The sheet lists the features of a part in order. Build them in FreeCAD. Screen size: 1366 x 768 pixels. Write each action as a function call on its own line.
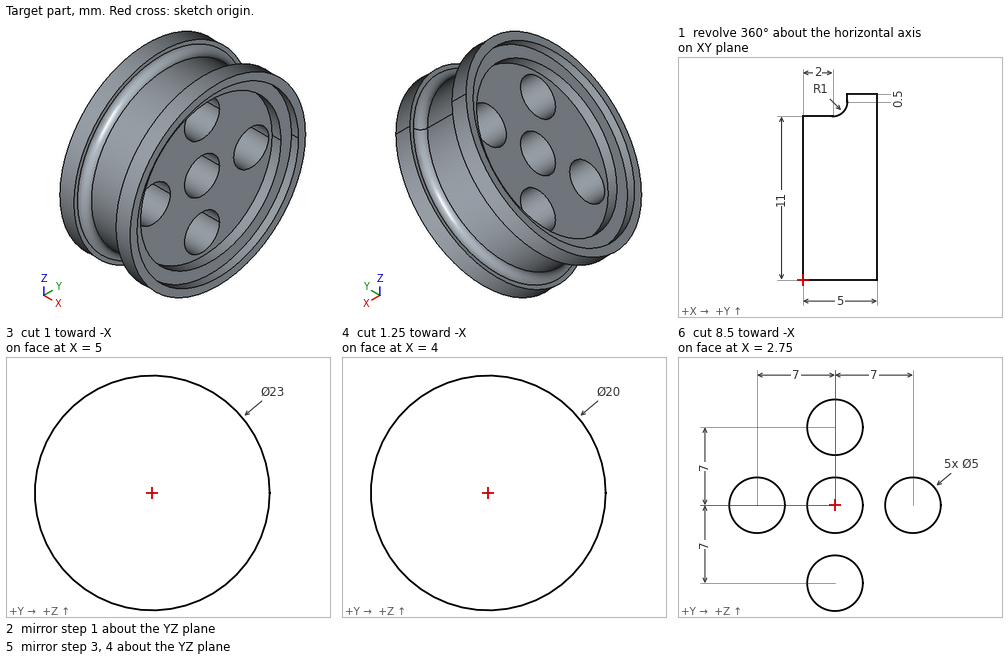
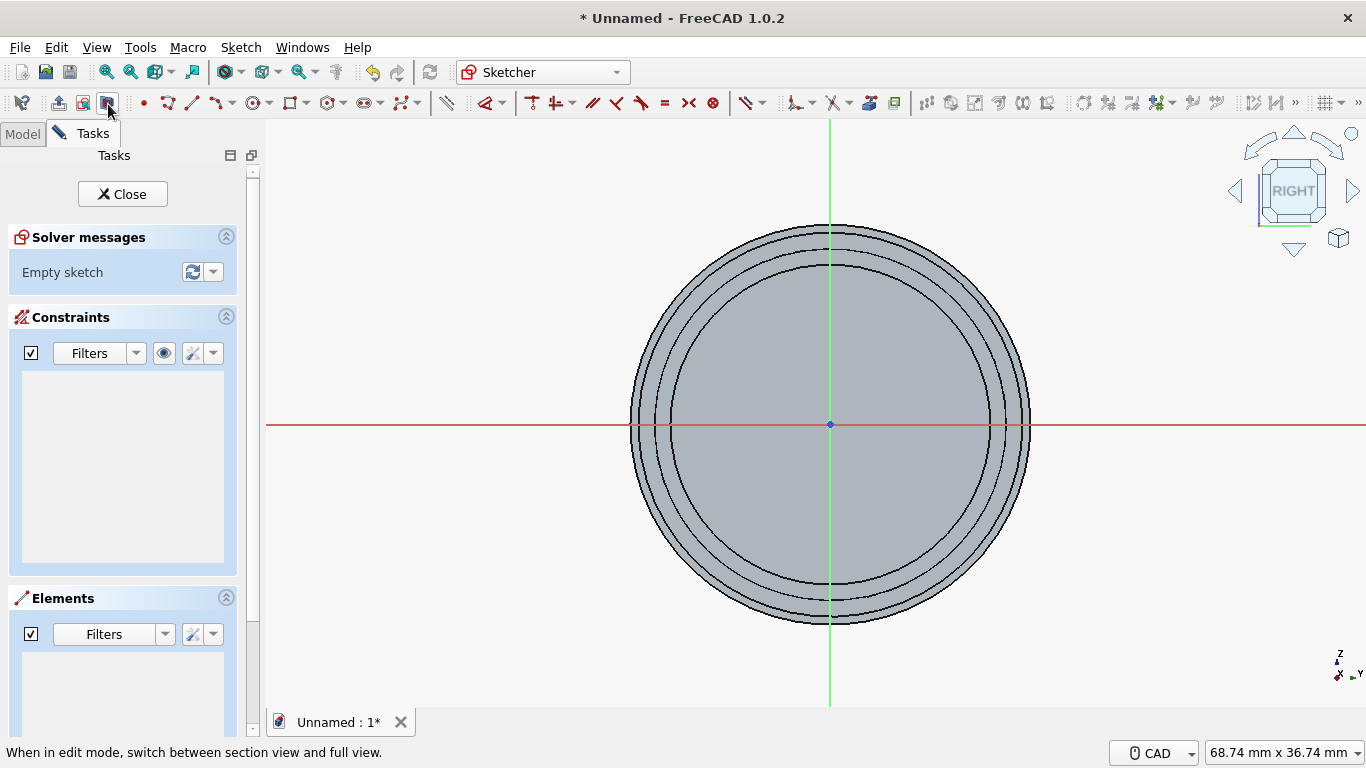
click(254, 104)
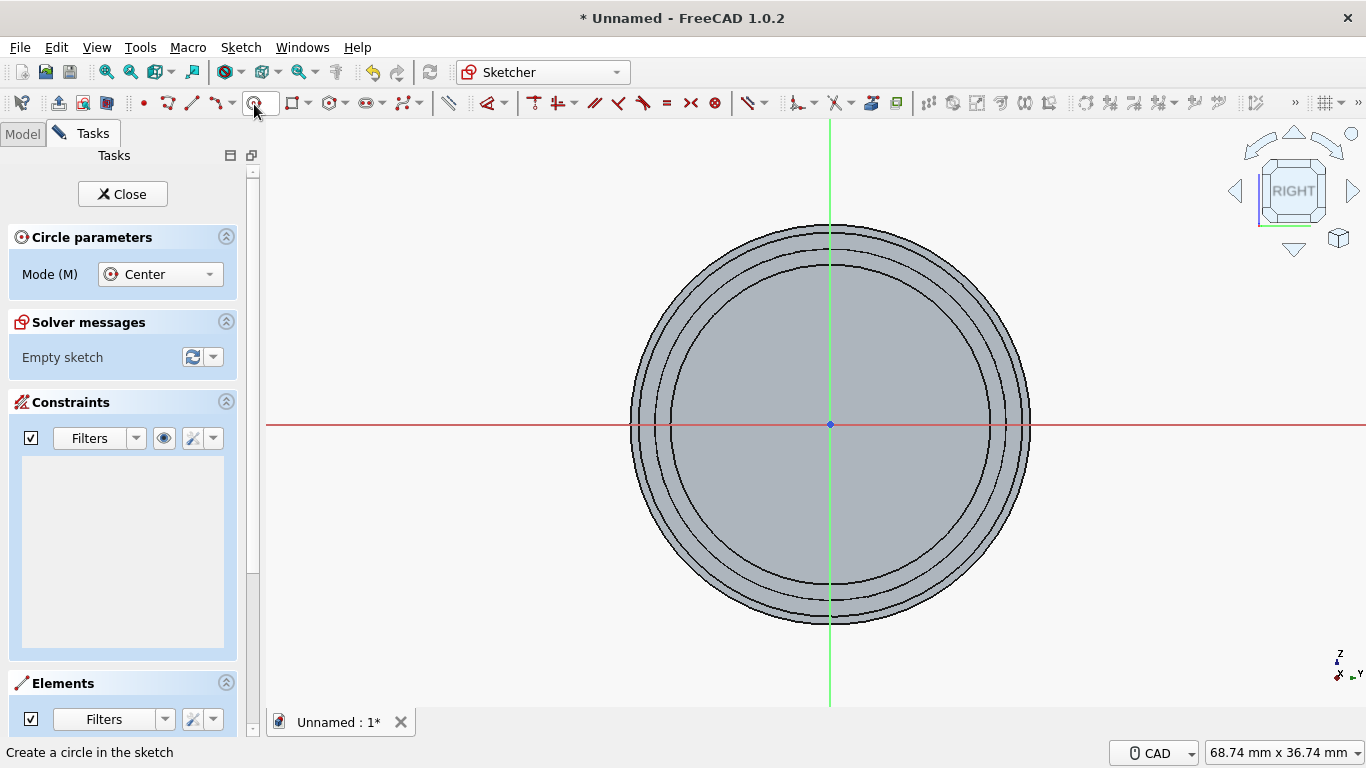
click(942, 425)
click(971, 396)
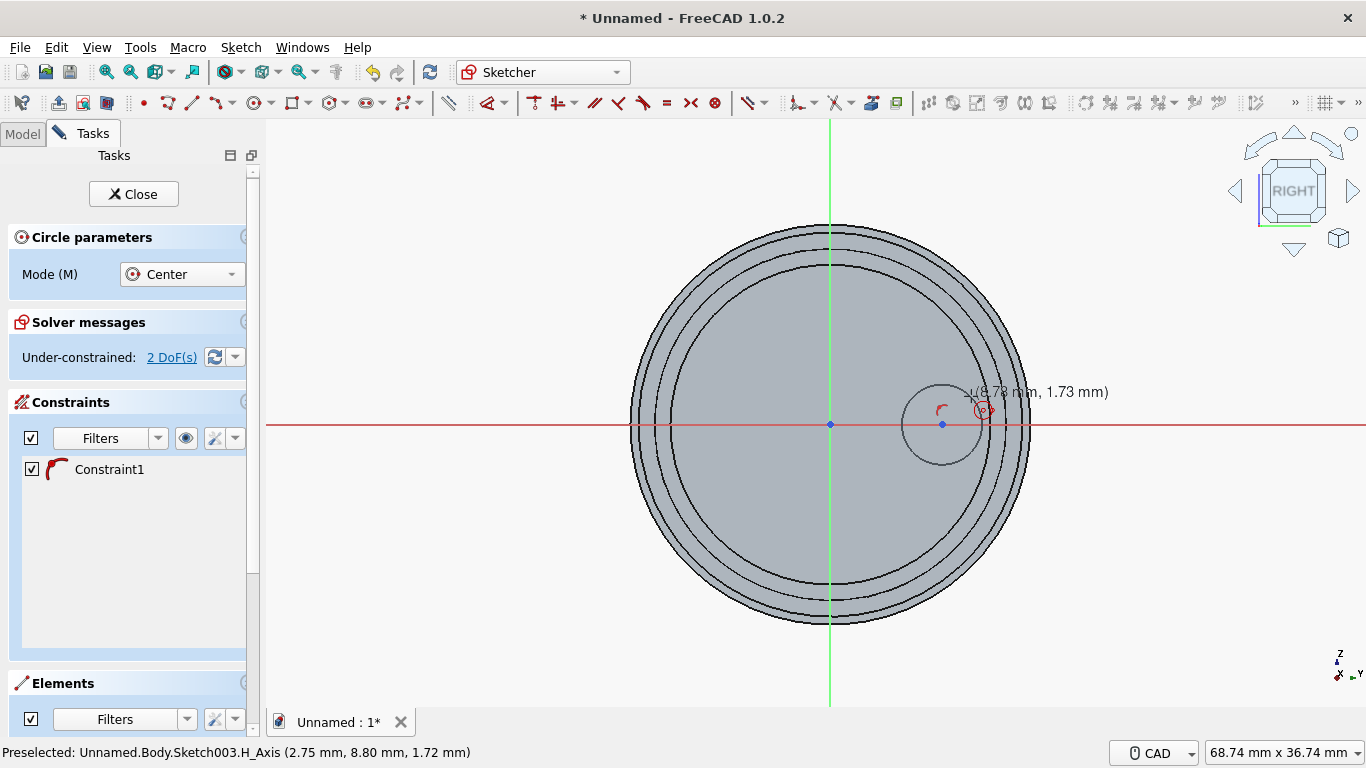
click(830, 537)
click(859, 508)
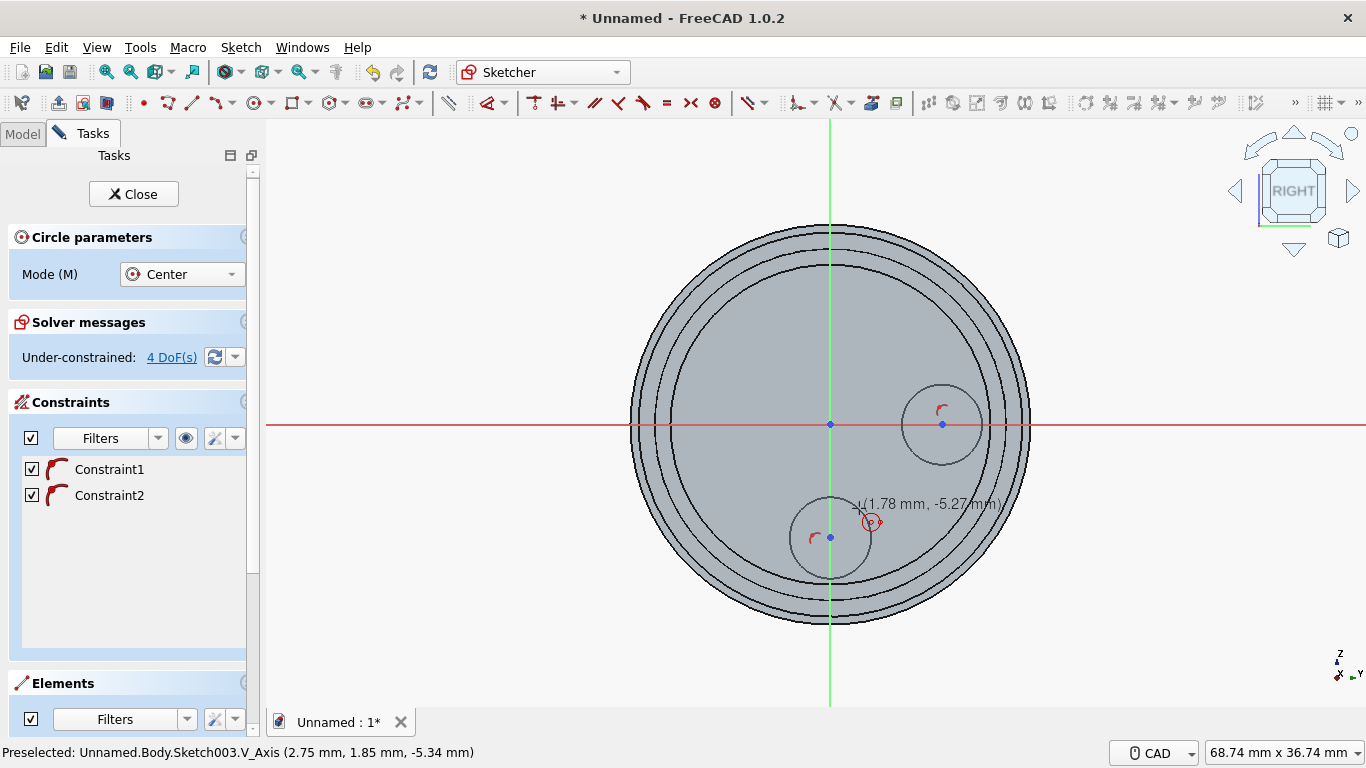
click(718, 425)
click(747, 396)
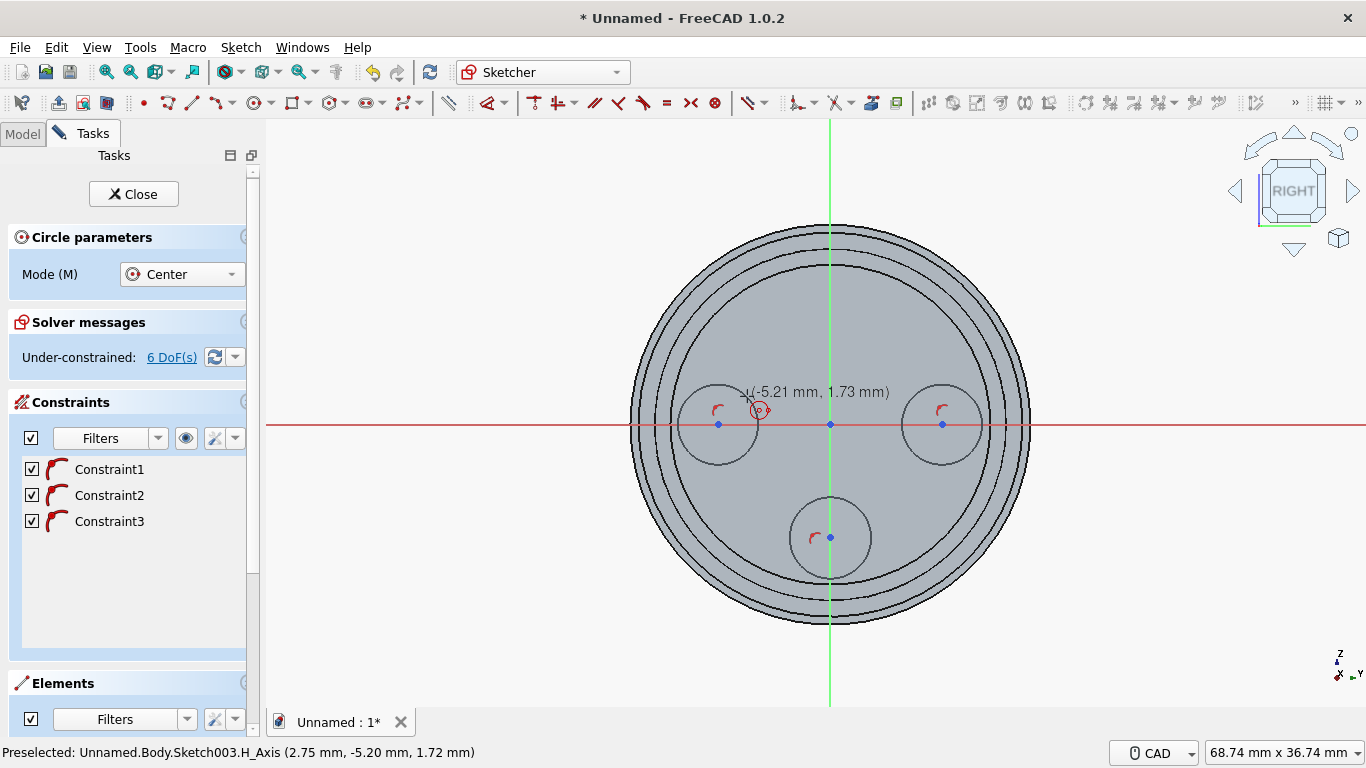
click(830, 313)
click(859, 284)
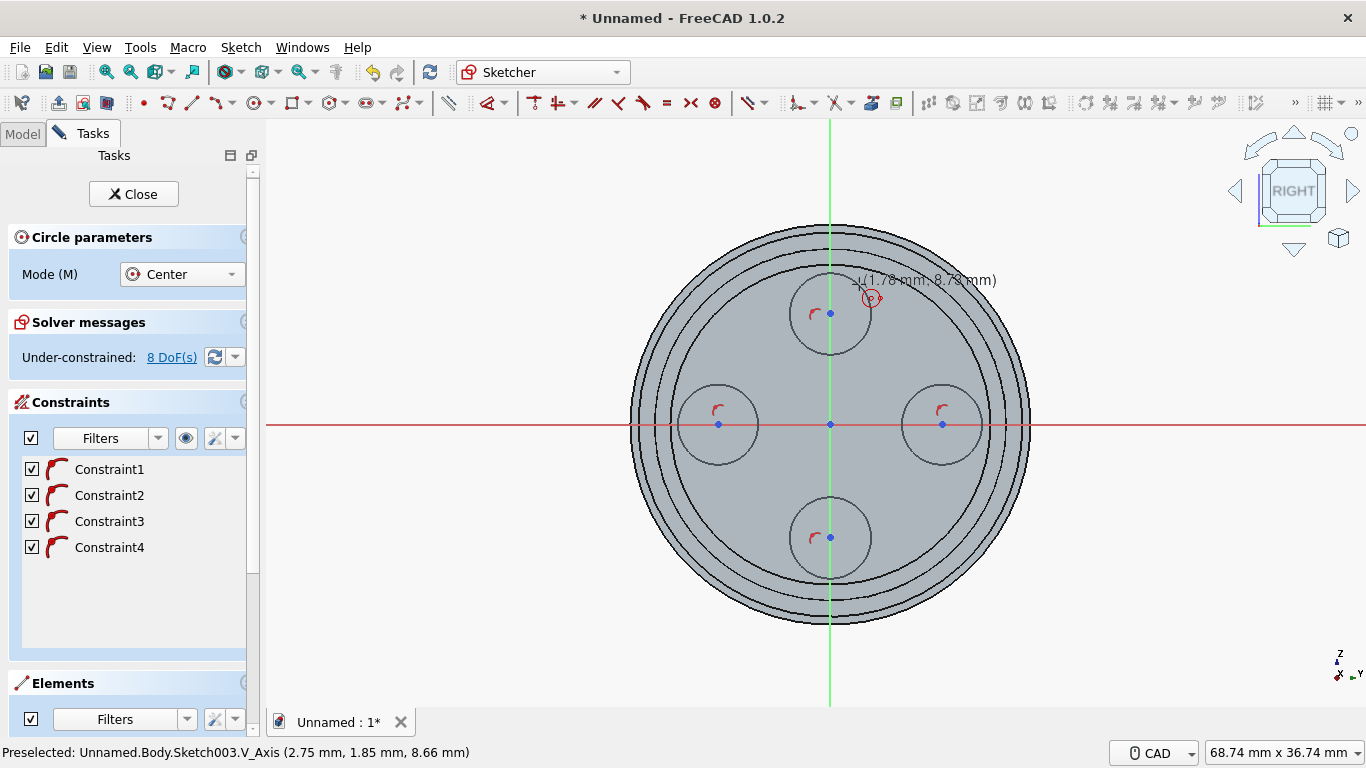
click(830, 425)
click(859, 396)
key(Escape)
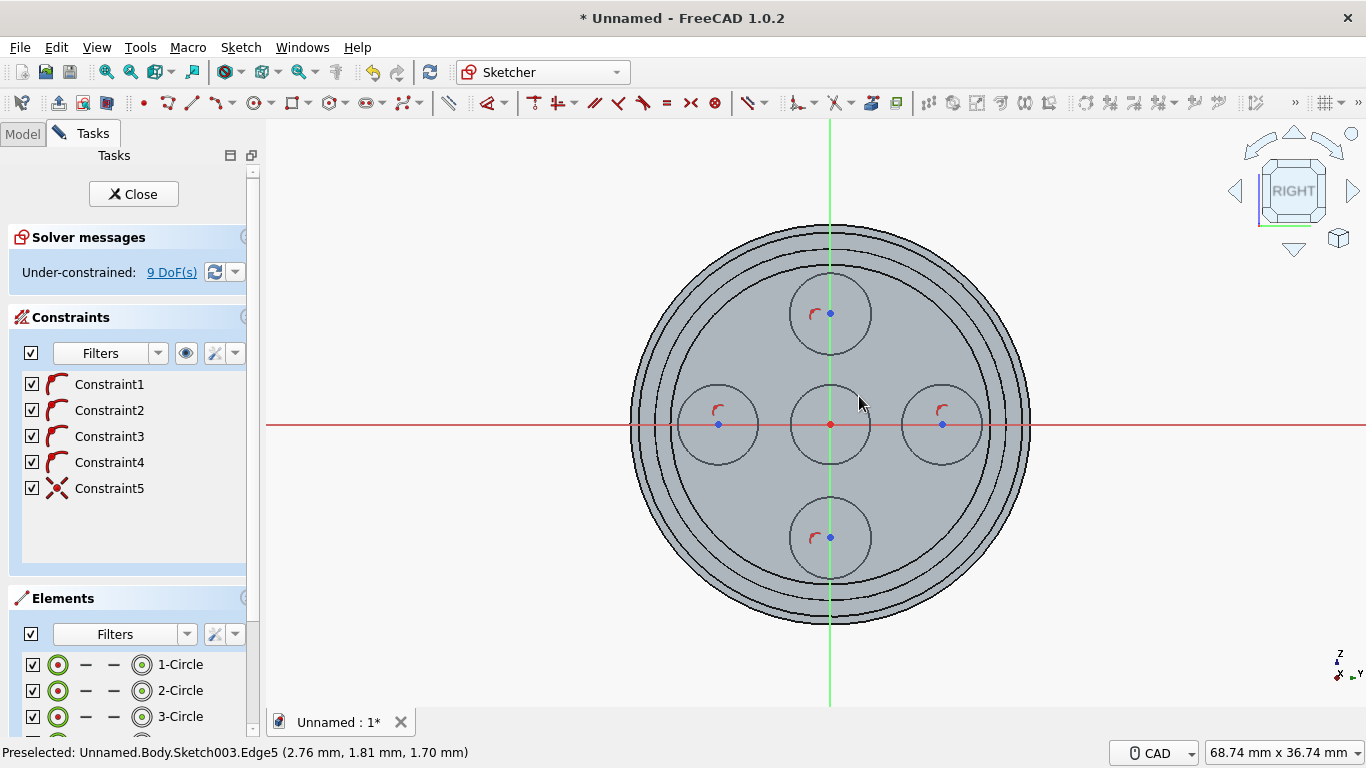
click(970, 396)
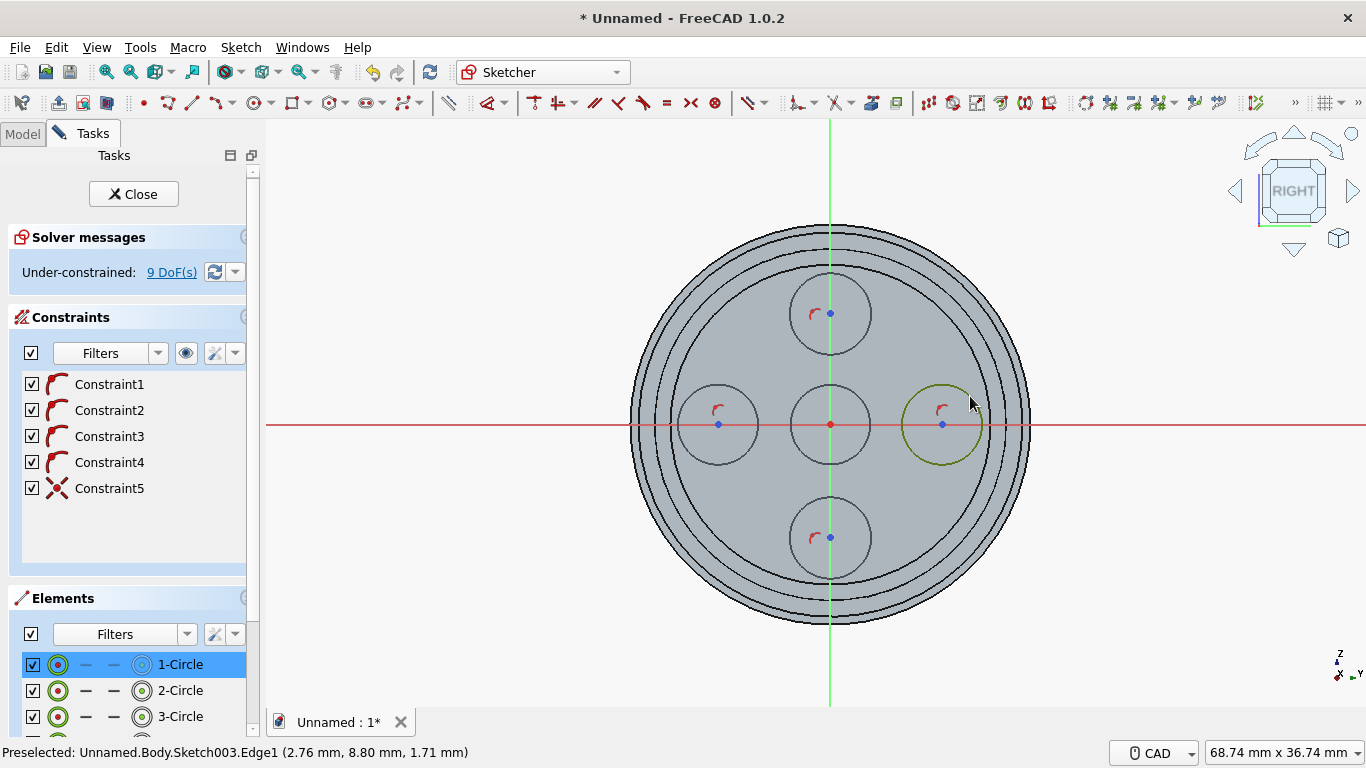
click(859, 509)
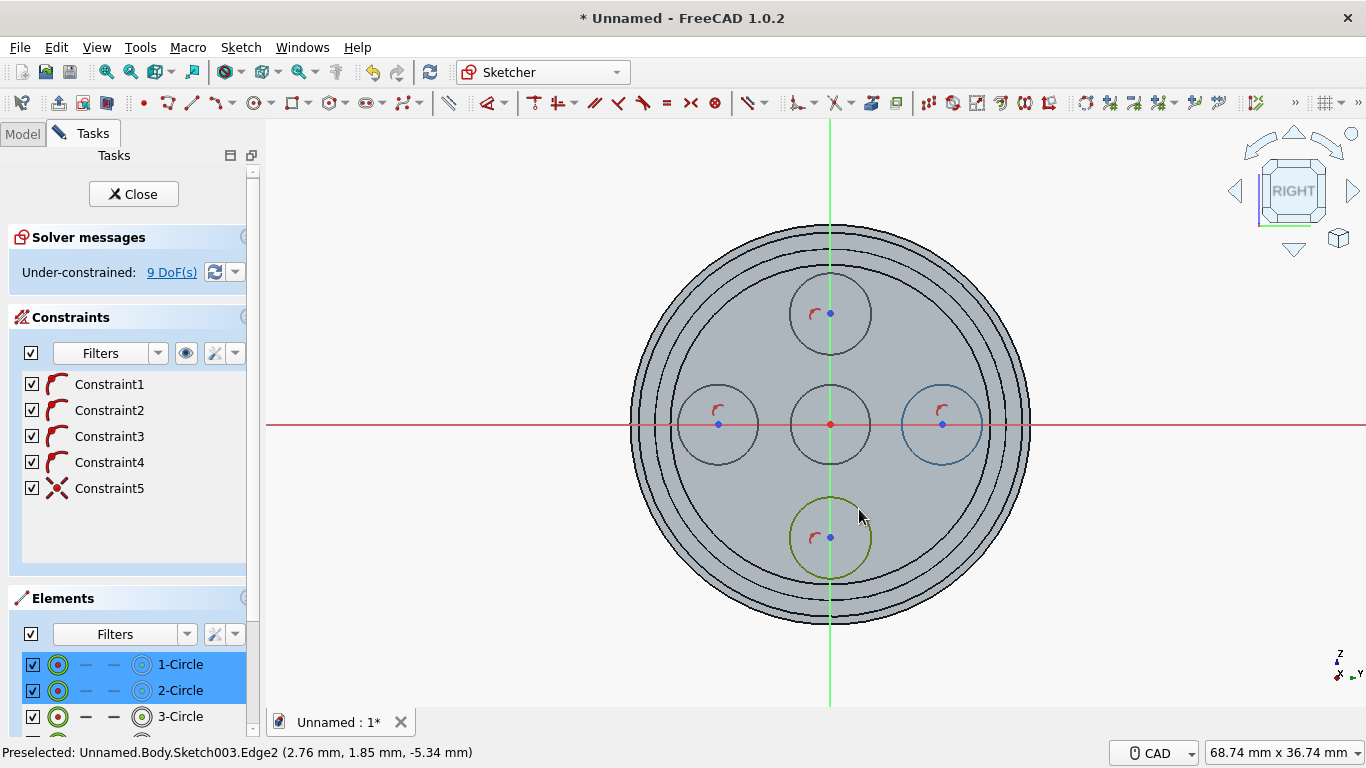
click(746, 396)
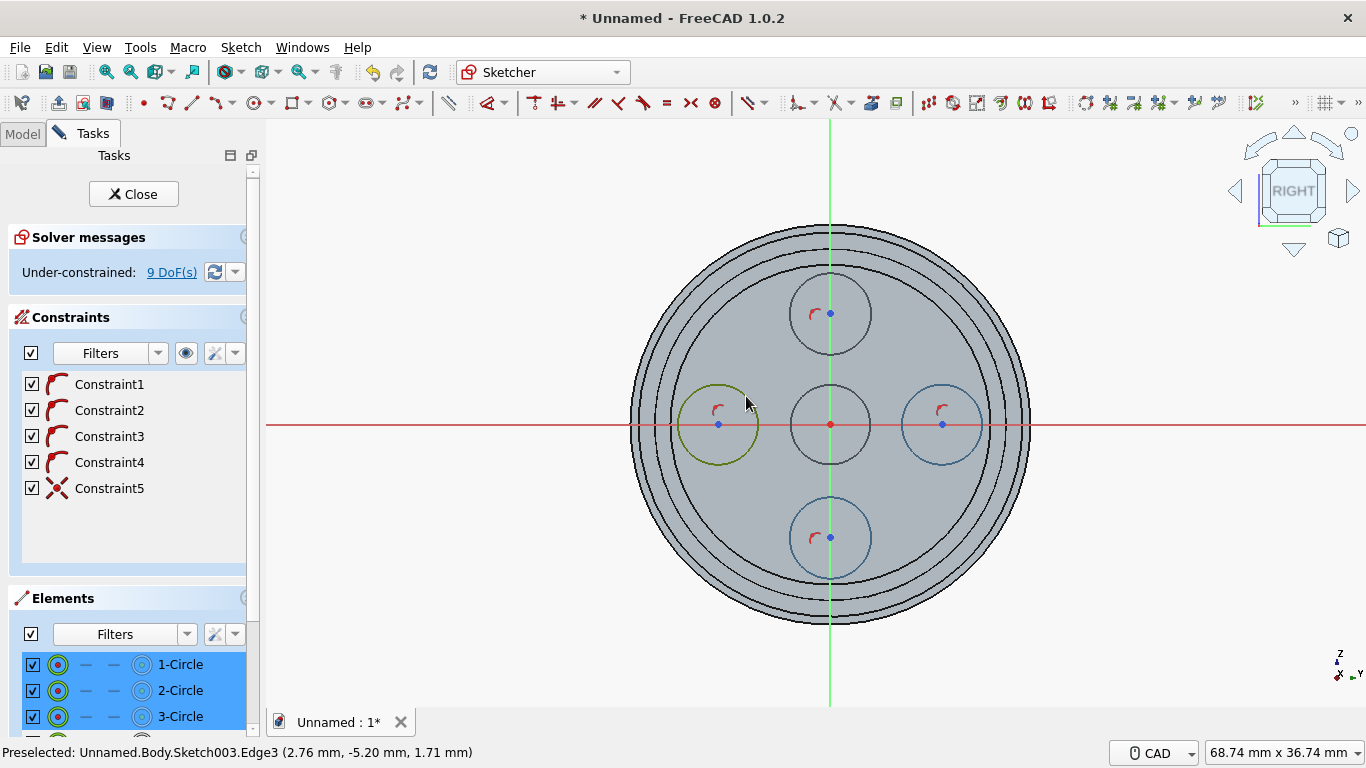
click(859, 285)